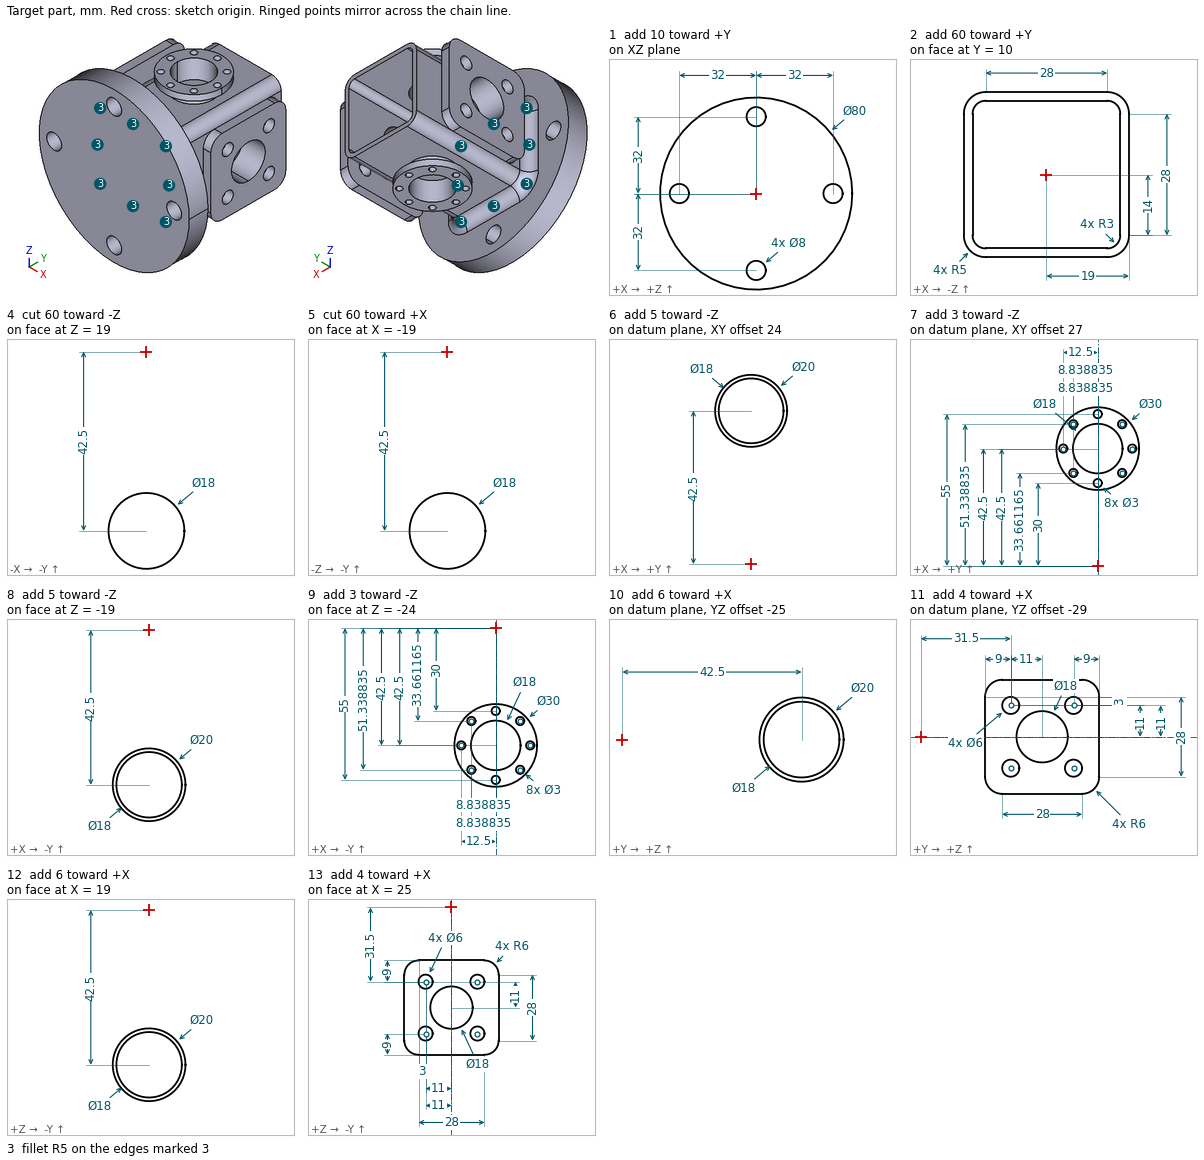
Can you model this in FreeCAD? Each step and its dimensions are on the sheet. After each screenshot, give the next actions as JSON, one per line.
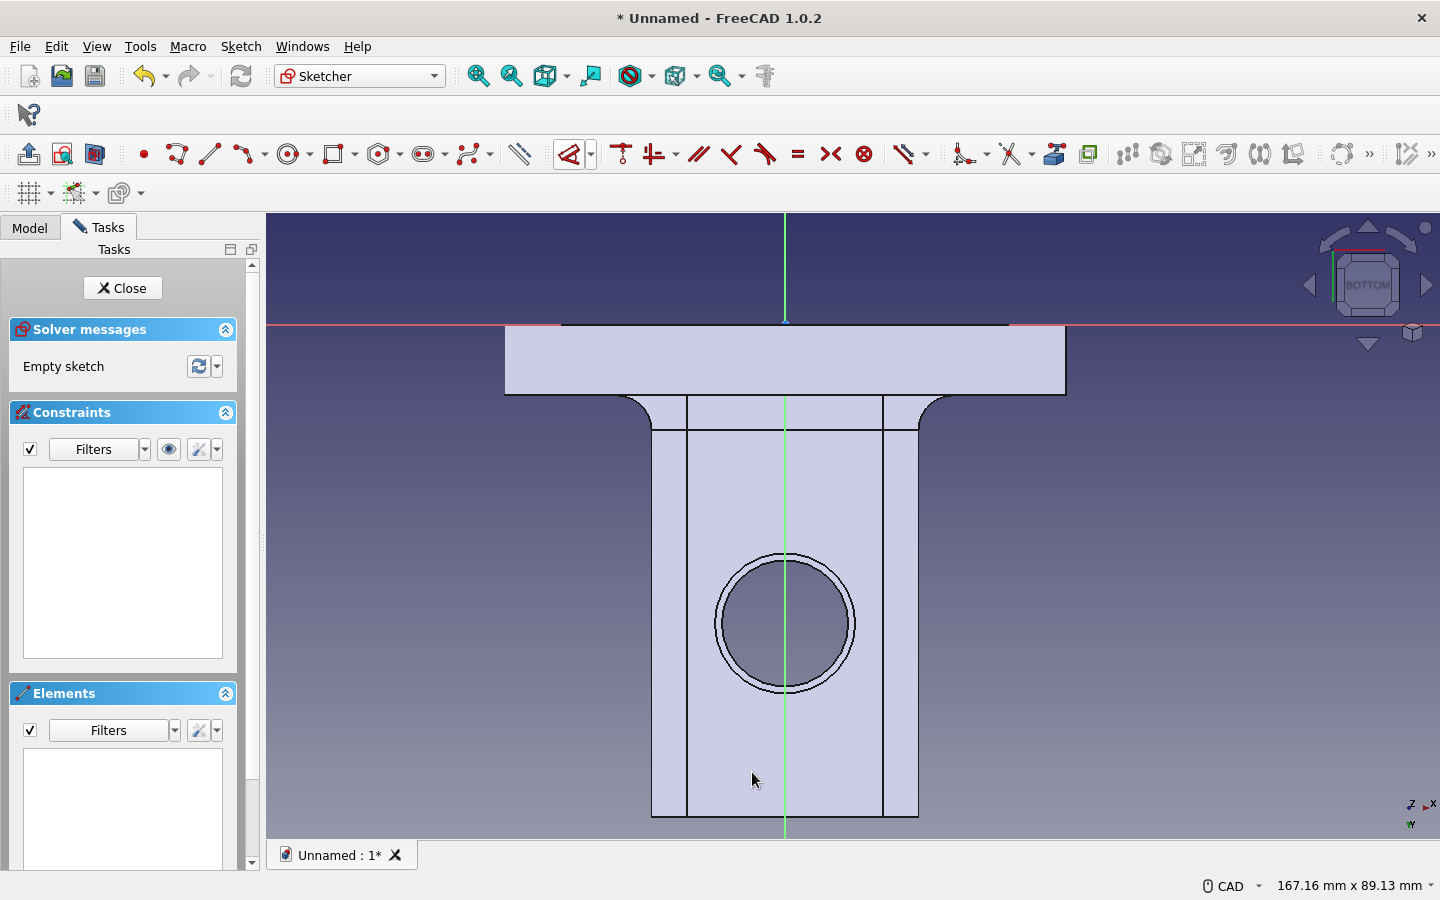
{"action": "left_click", "coordinate": [288, 154]}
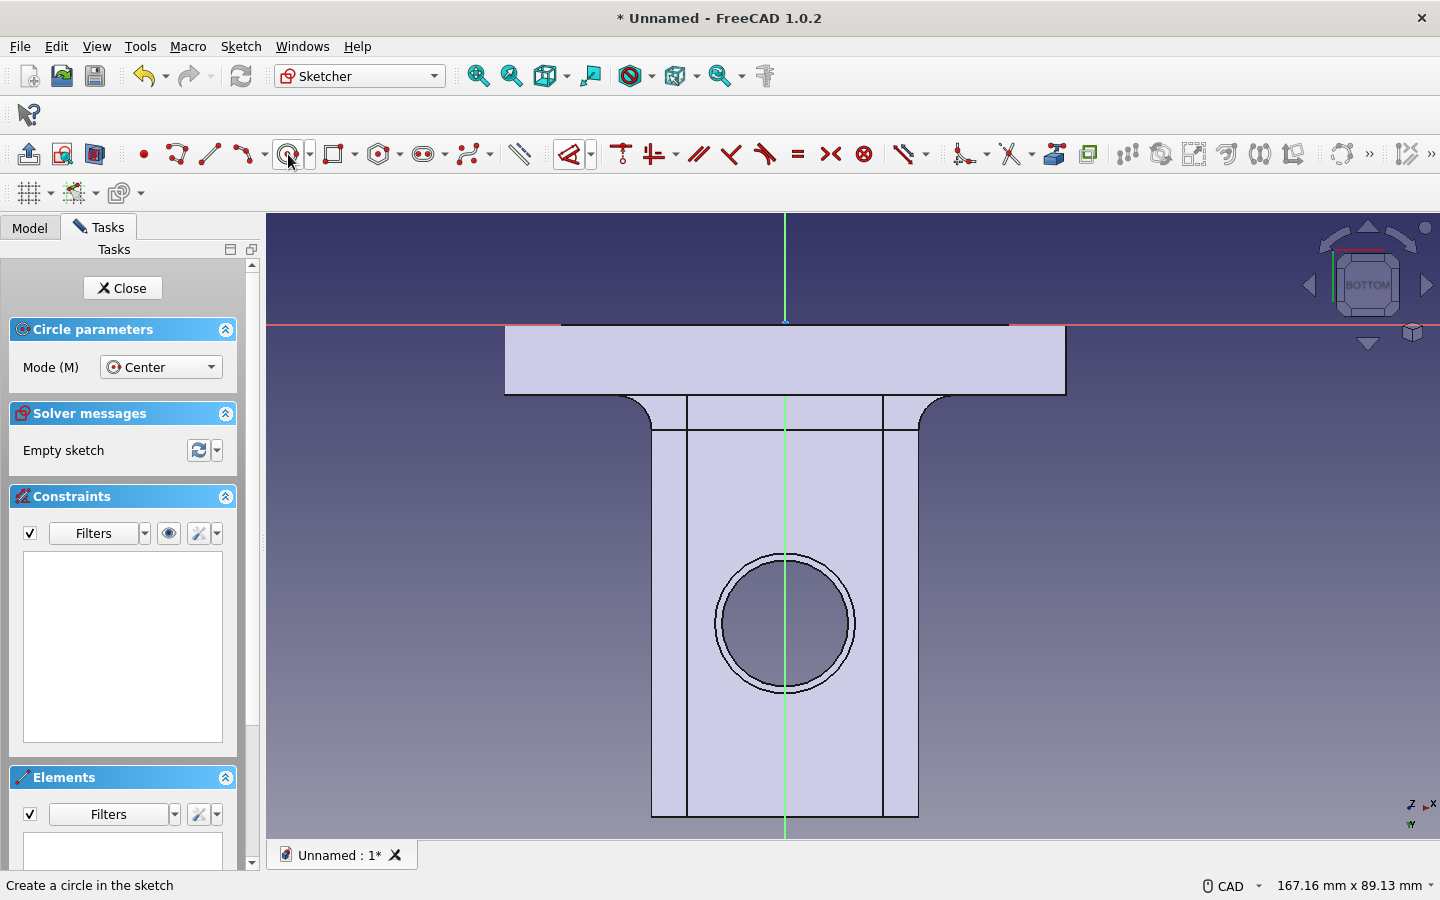
{"action": "left_click", "coordinate": [785, 623]}
{"action": "mouse_move", "coordinate": [860, 549]}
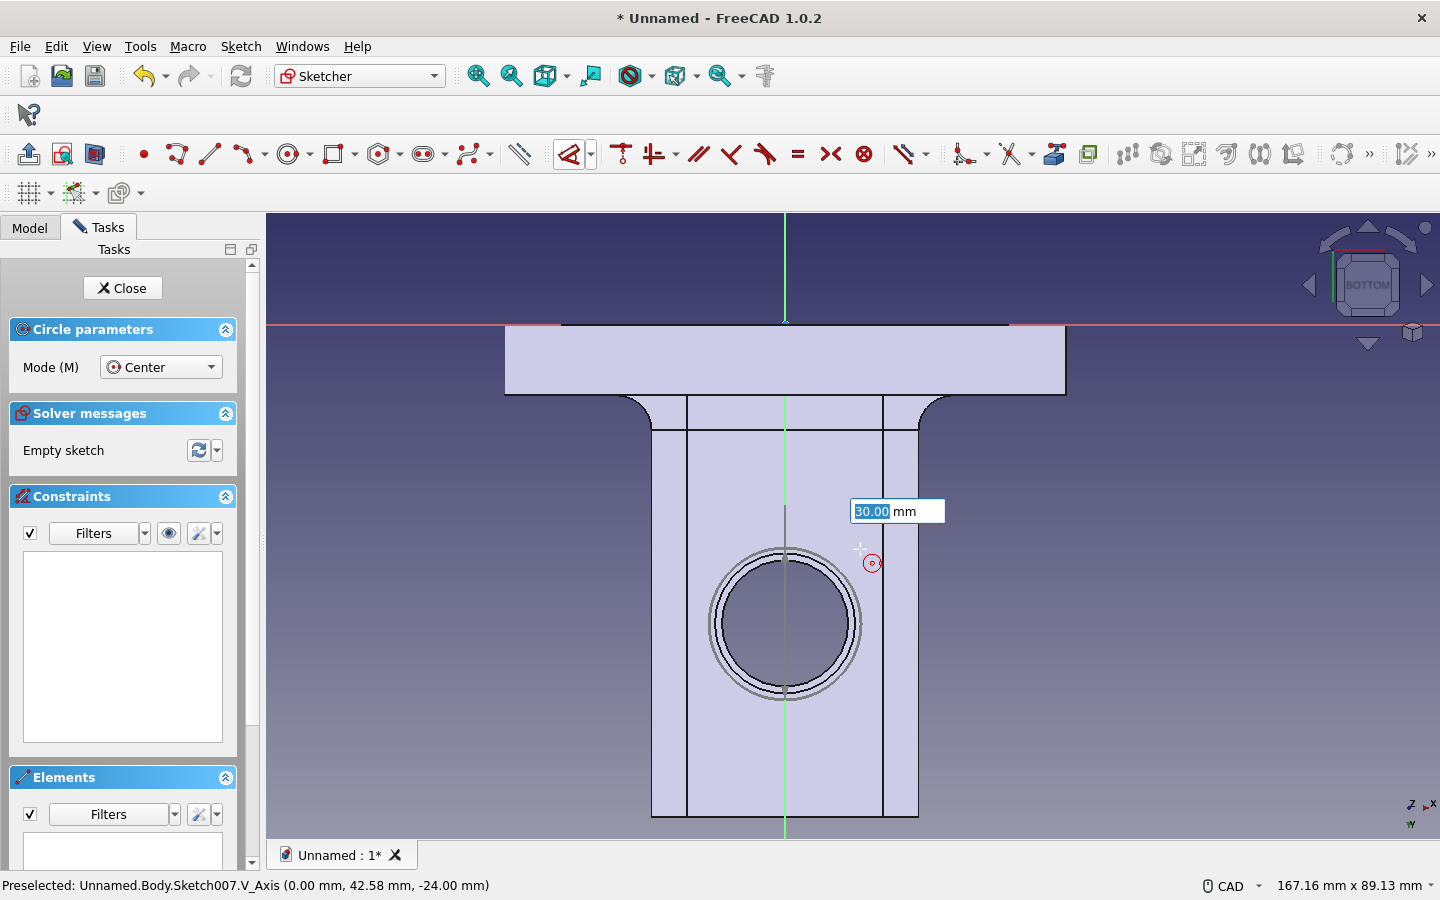
{"action": "type", "text": "30"}
{"action": "key", "text": "Return"}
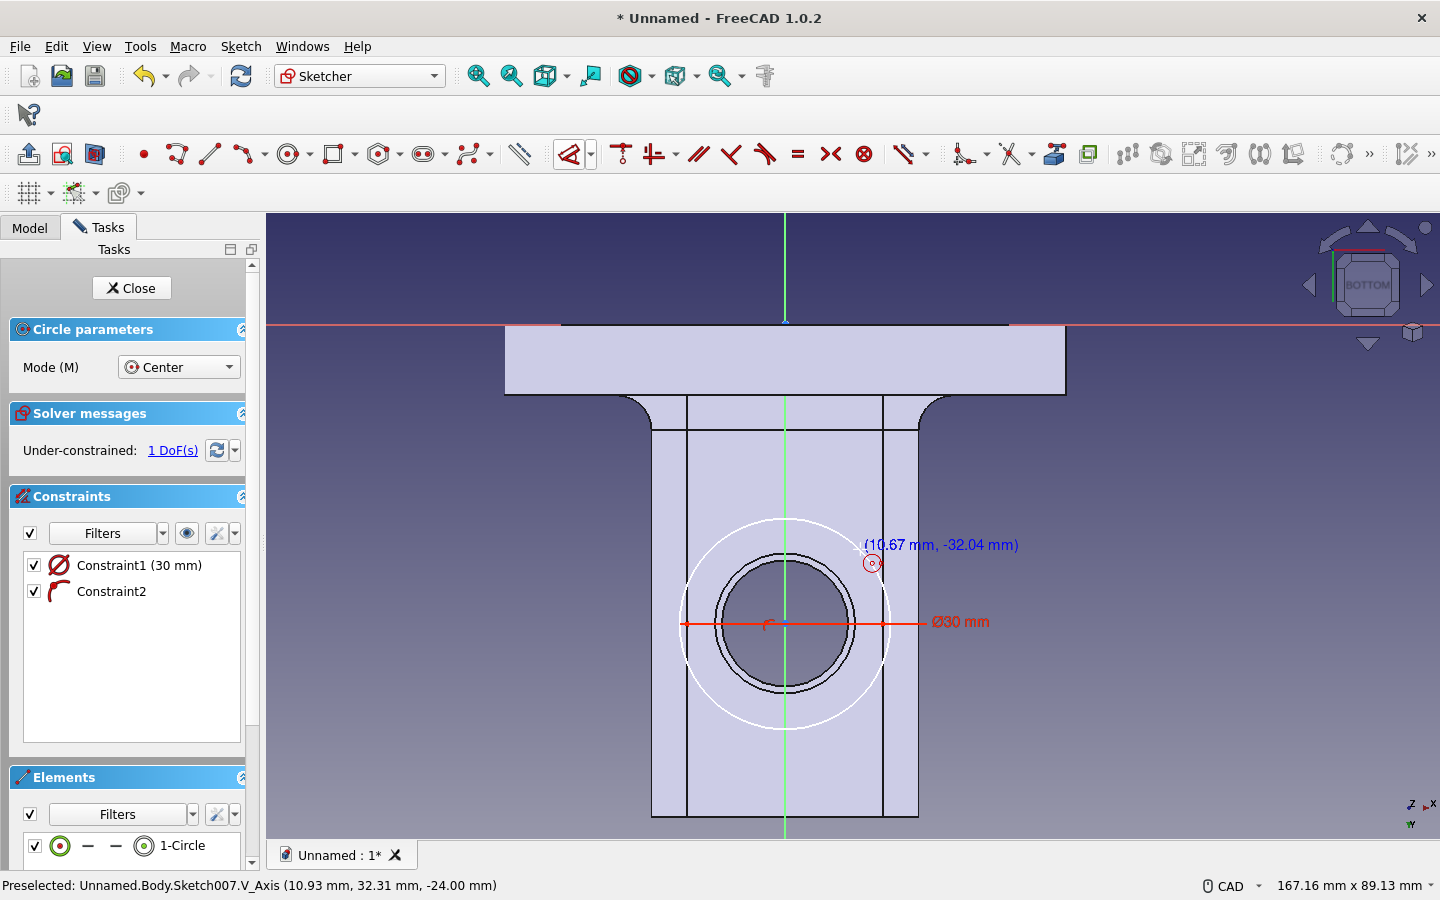
{"action": "scroll", "coordinate": [723, 686], "scroll_direction": "up", "scroll_amount": 4}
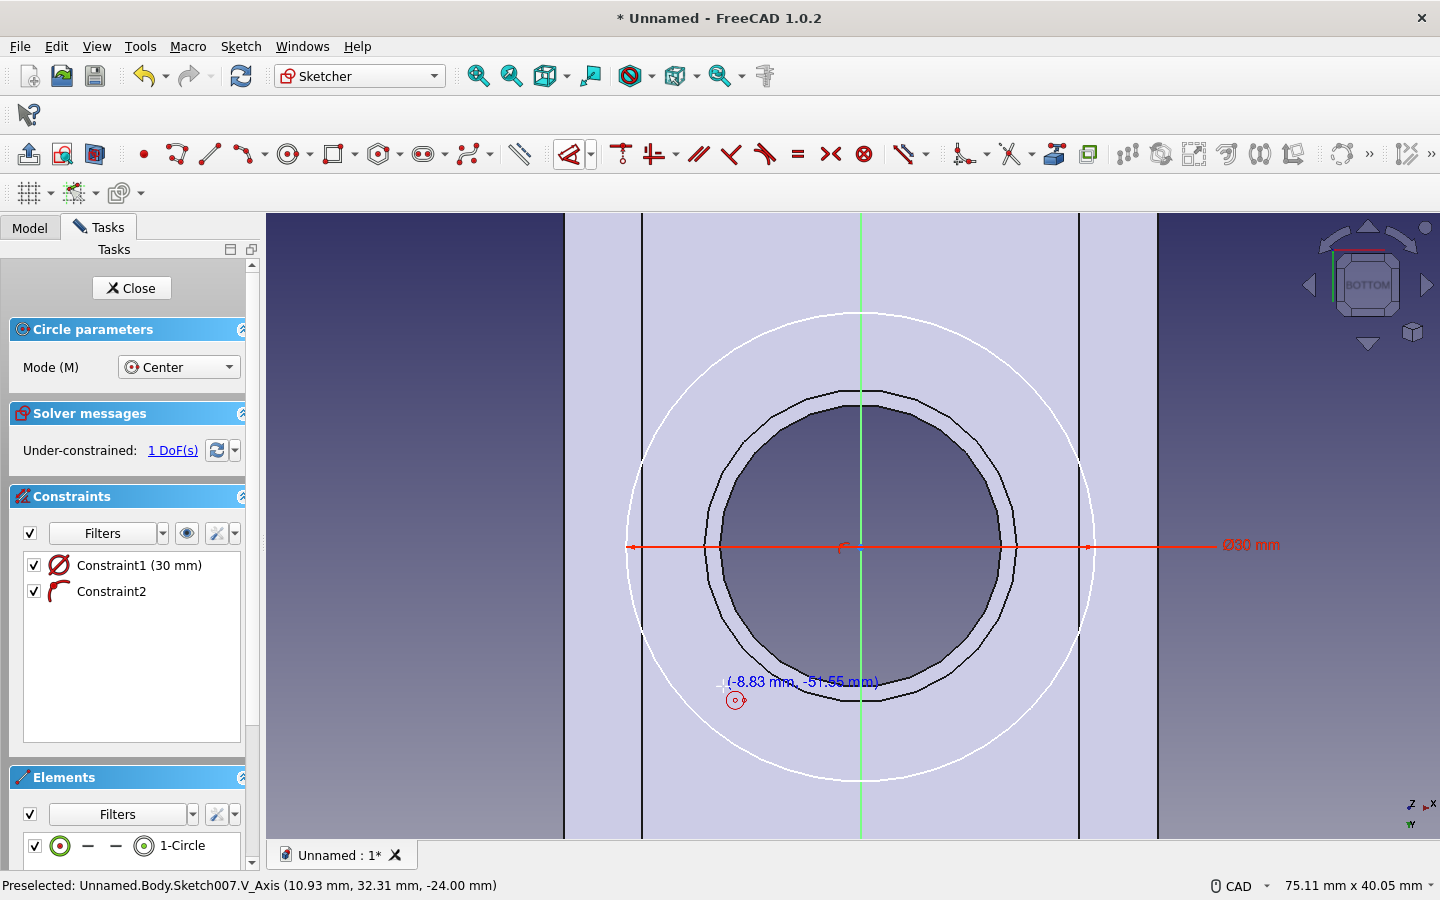
{"action": "left_click", "coordinate": [722, 684]}
{"action": "mouse_move", "coordinate": [739, 667]}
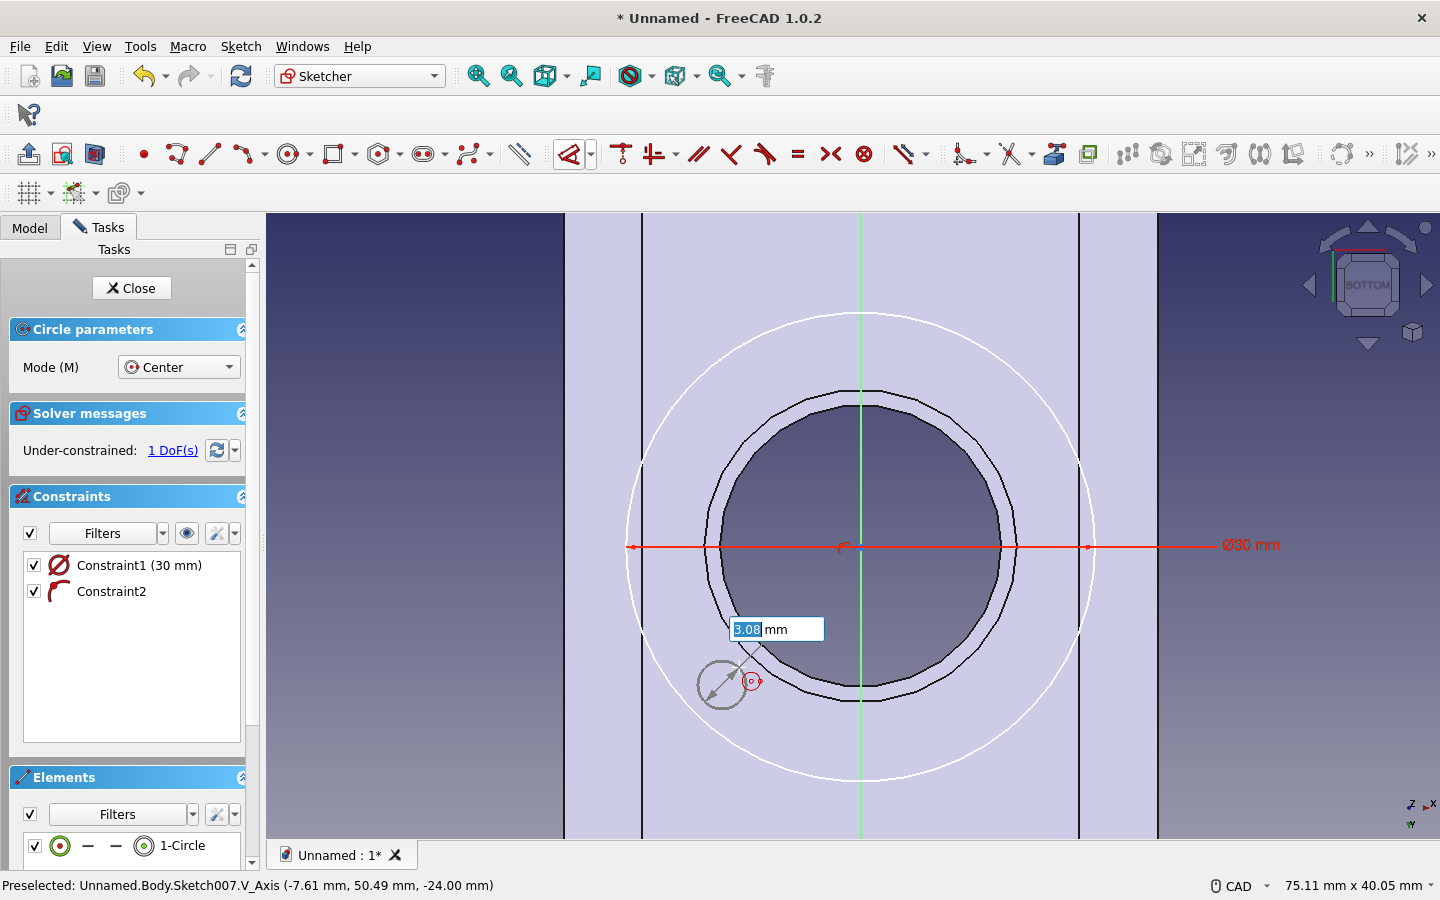
{"action": "type", "text": "3"}
{"action": "key", "text": "Return"}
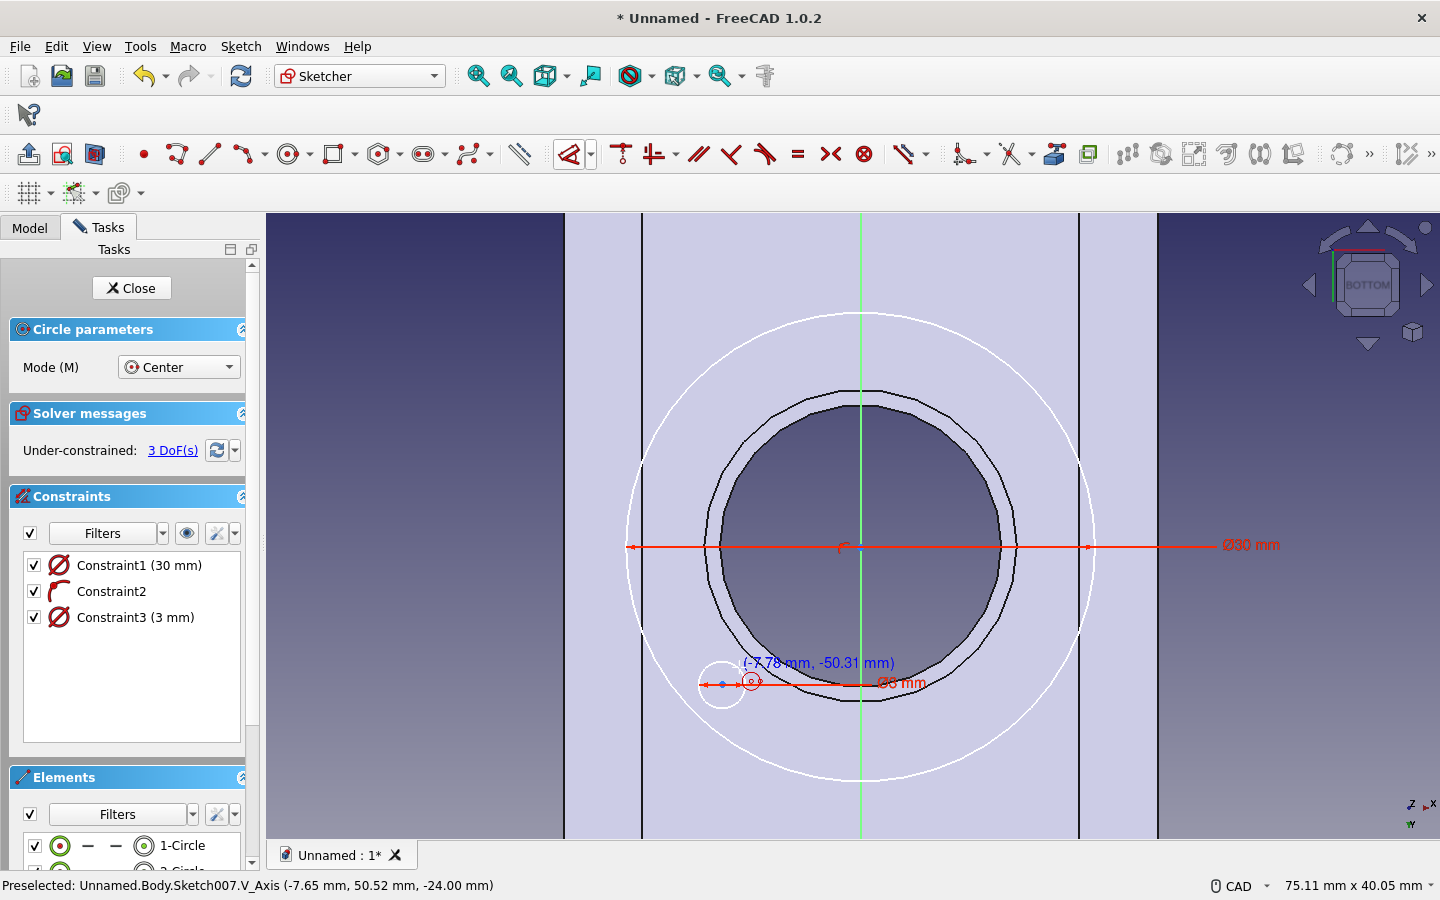
{"action": "left_click", "coordinate": [861, 741]}
{"action": "mouse_move", "coordinate": [877, 725]}